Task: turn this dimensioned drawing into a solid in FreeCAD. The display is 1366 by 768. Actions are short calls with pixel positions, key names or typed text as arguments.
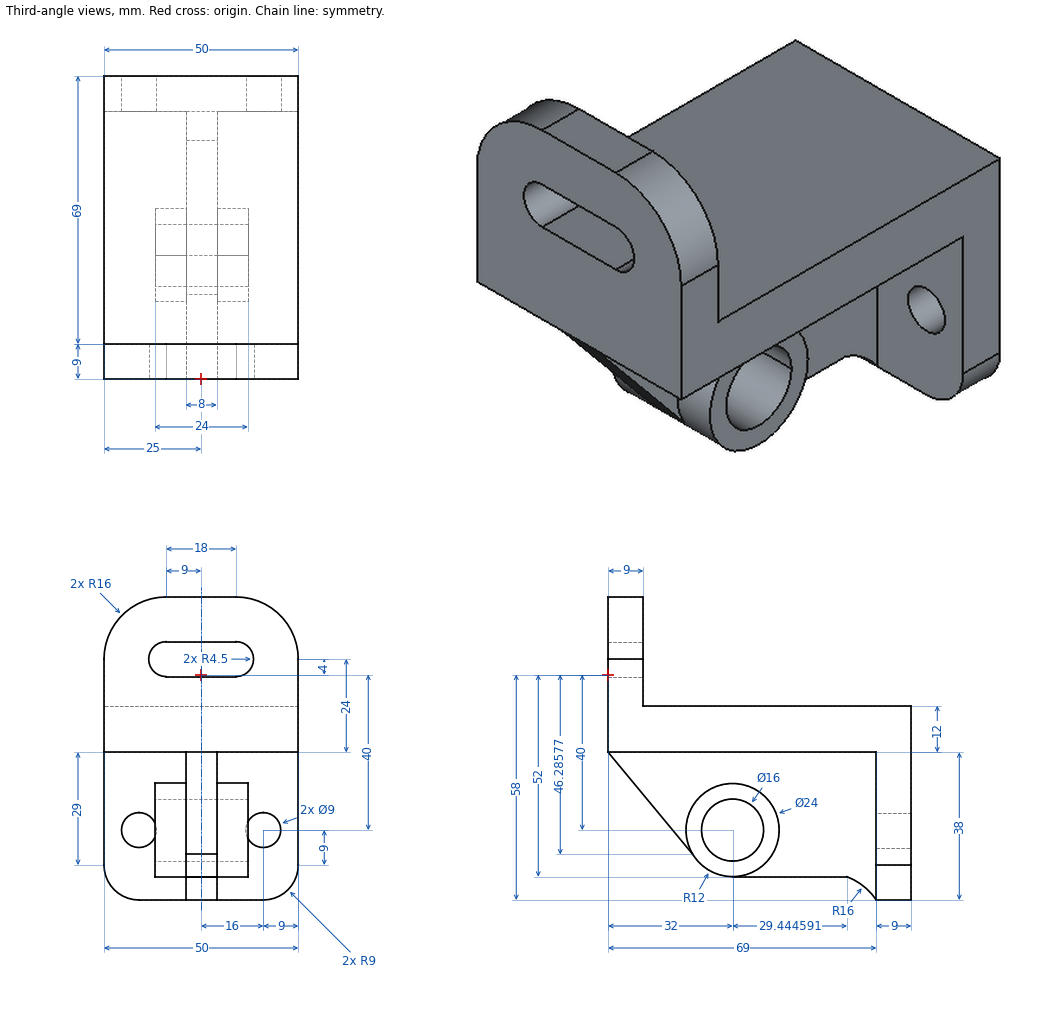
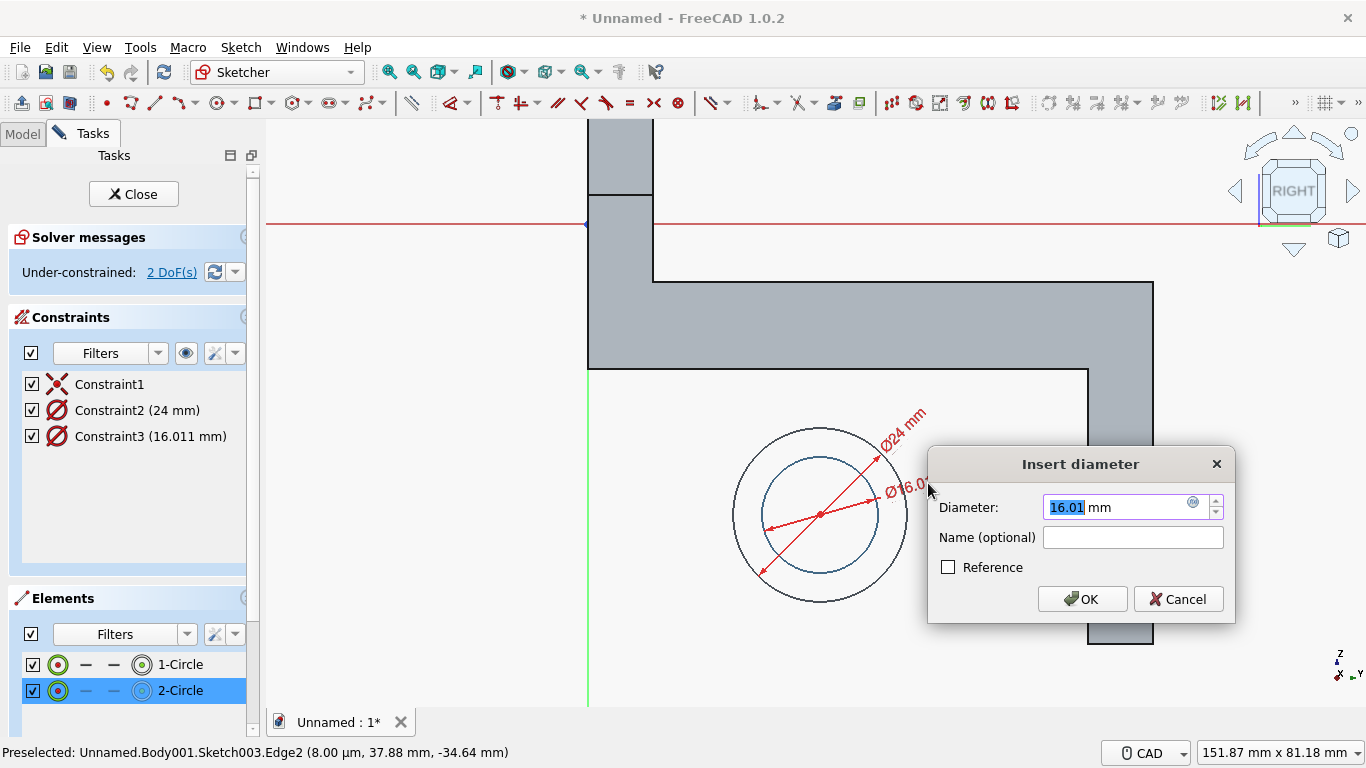
text(16)
key(Return)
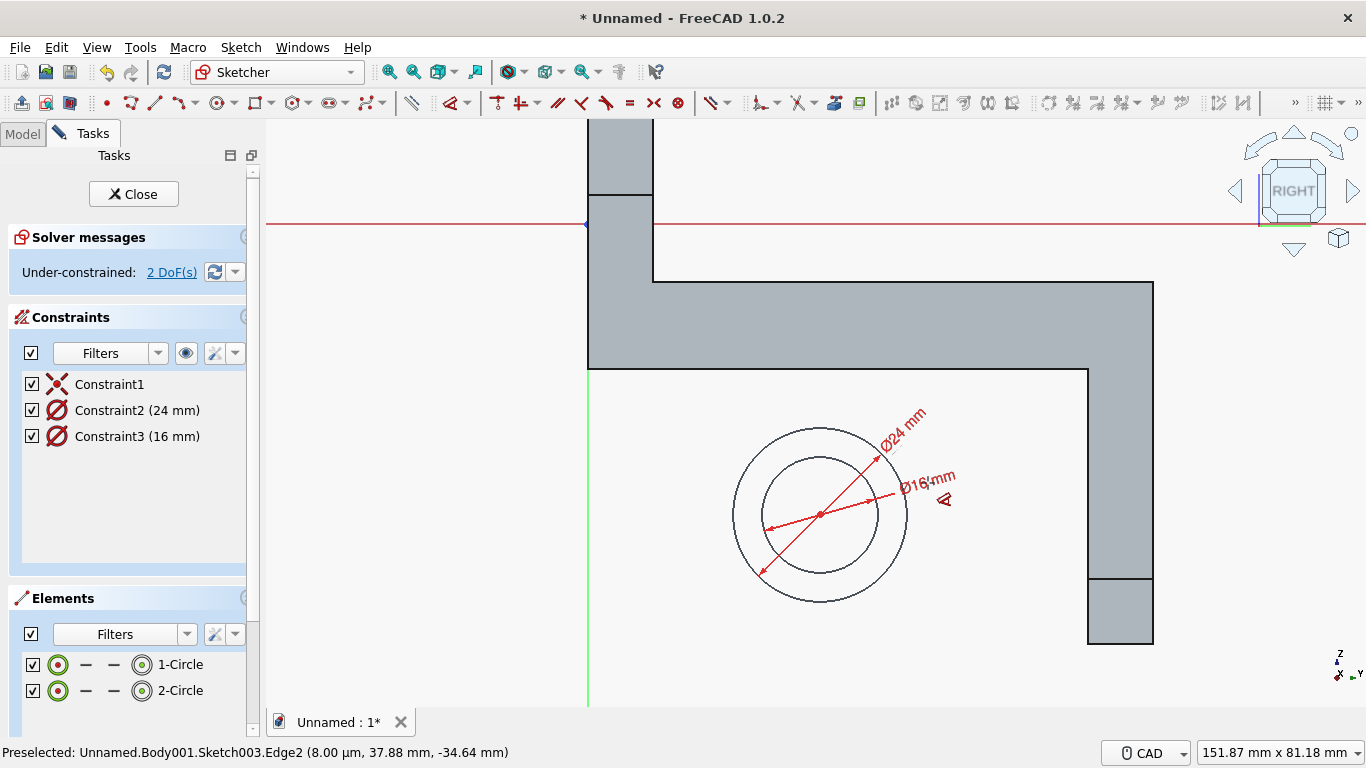
click(820, 515)
click(704, 190)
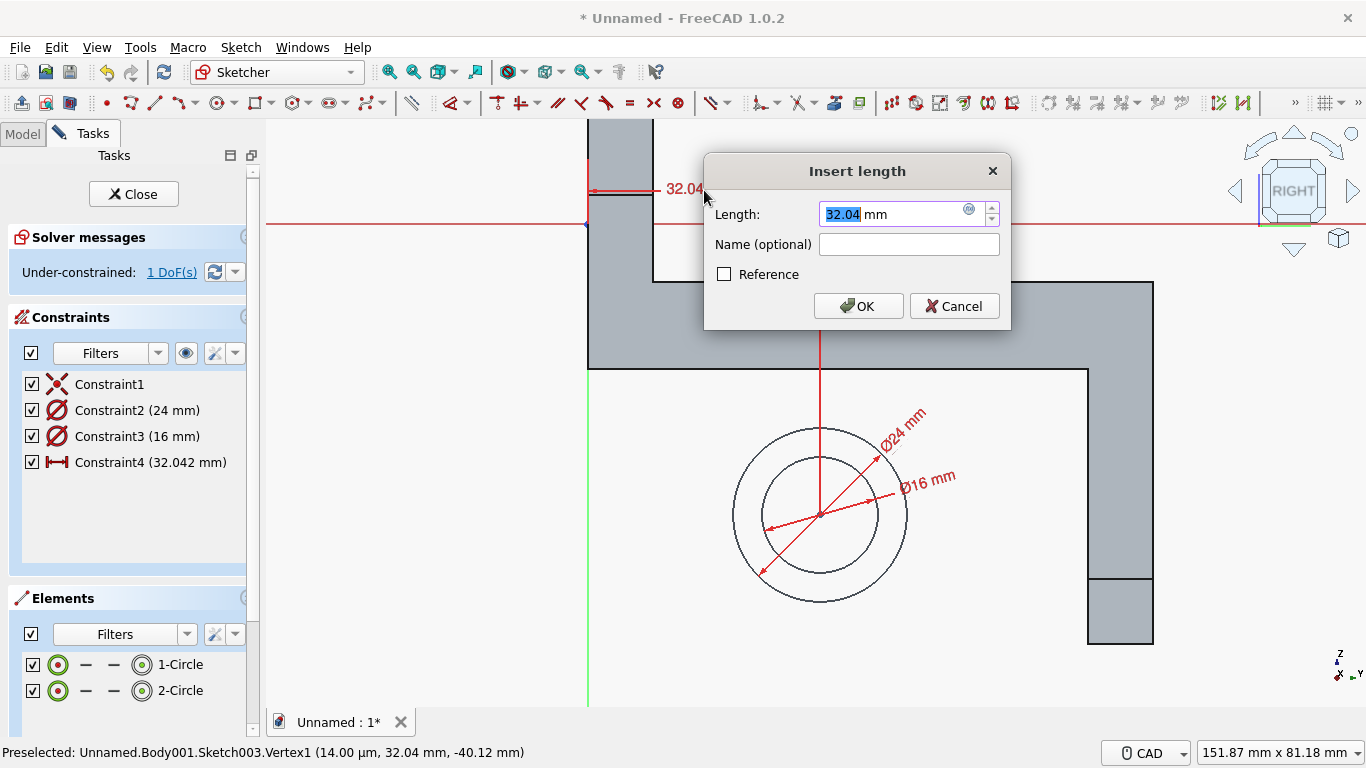
text(32)
key(Return)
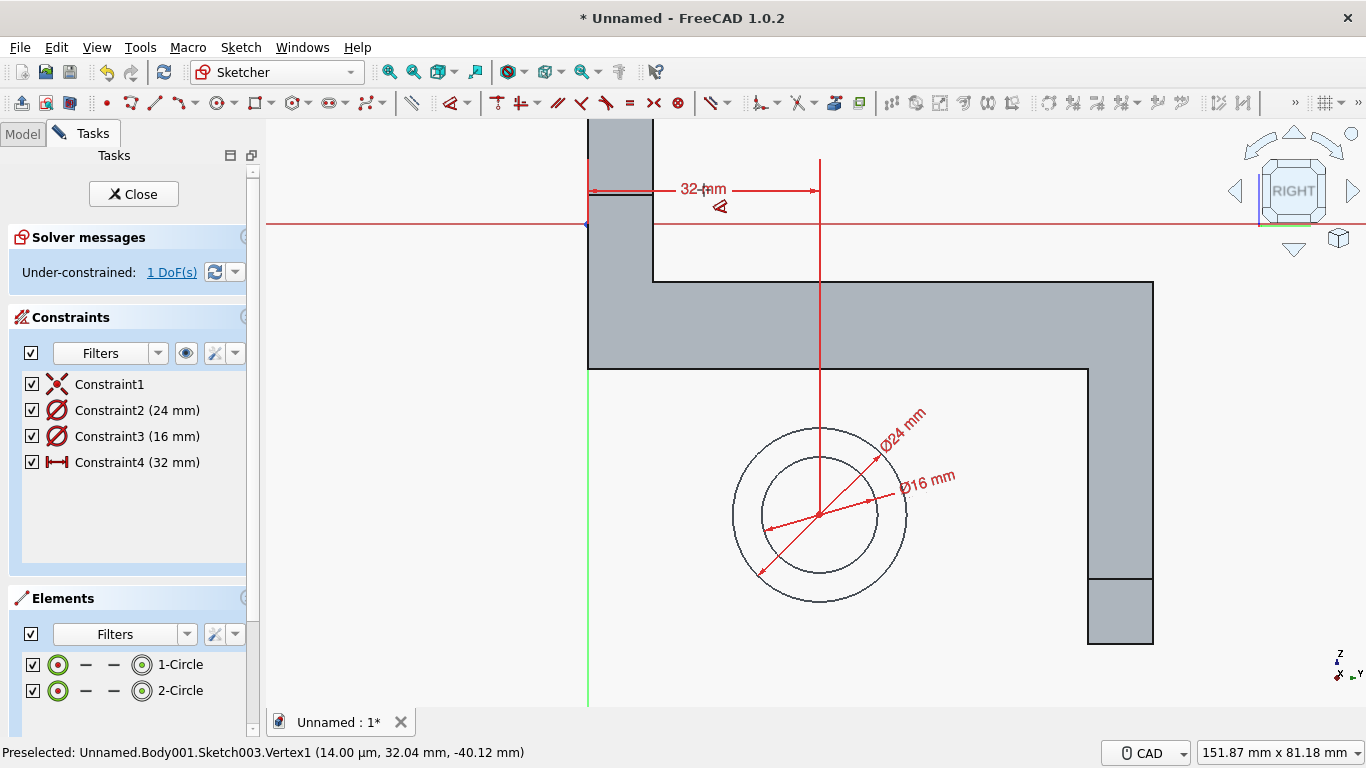
click(820, 515)
click(554, 370)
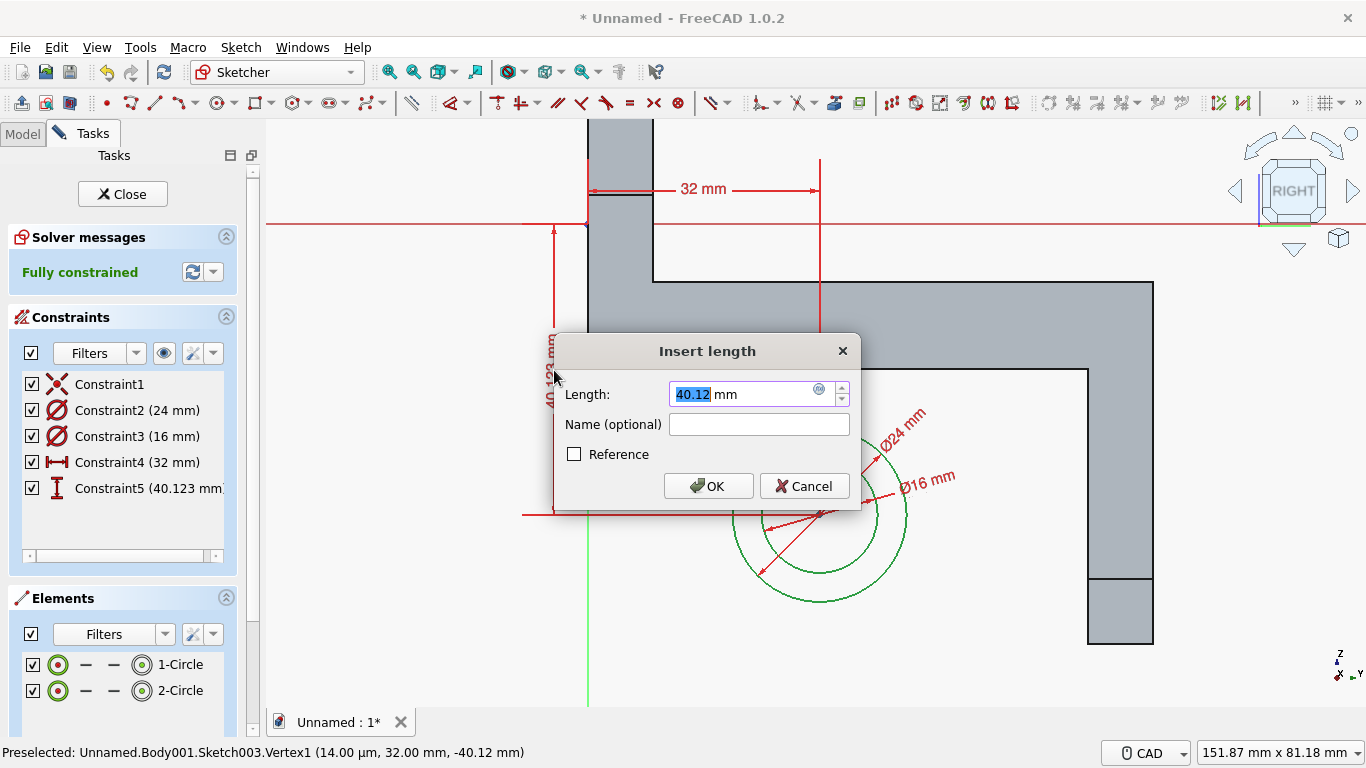
text(40)
key(Return)
key(Escape)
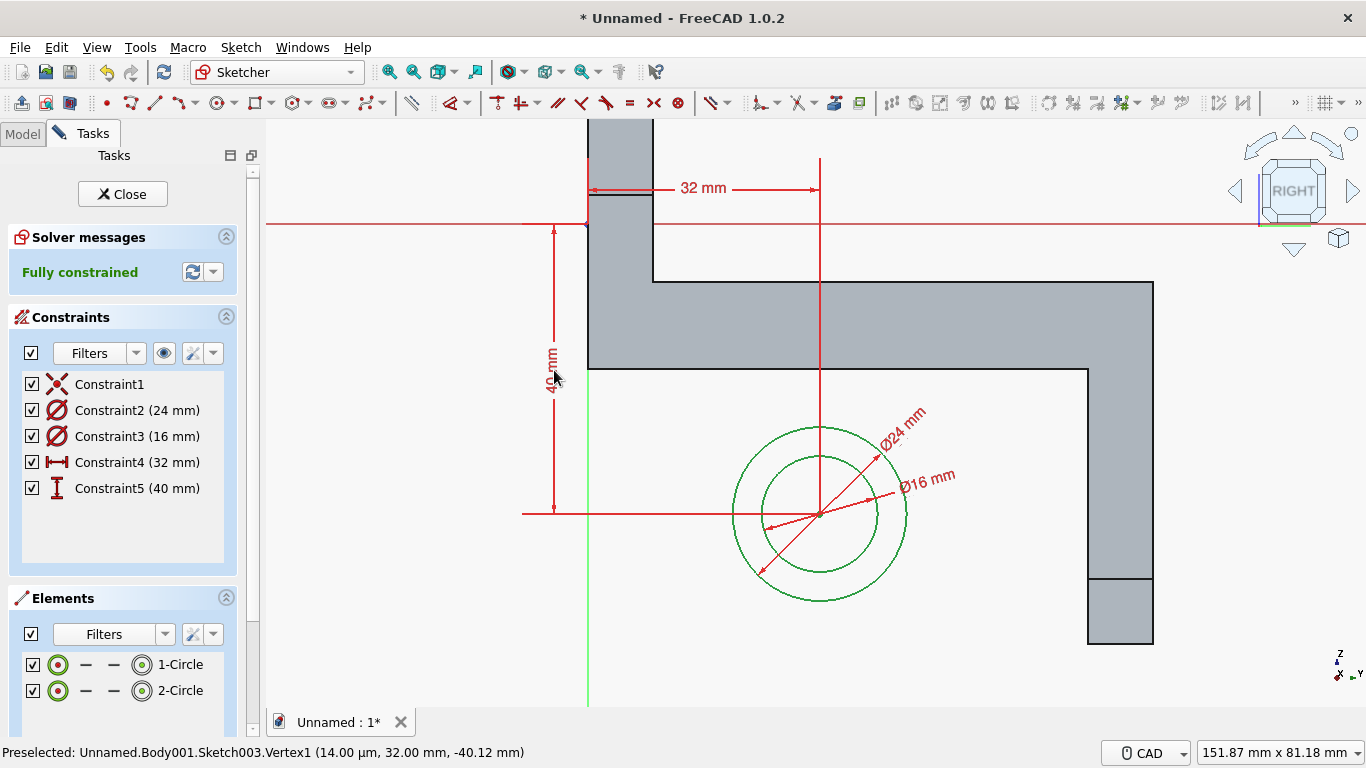
click(123, 194)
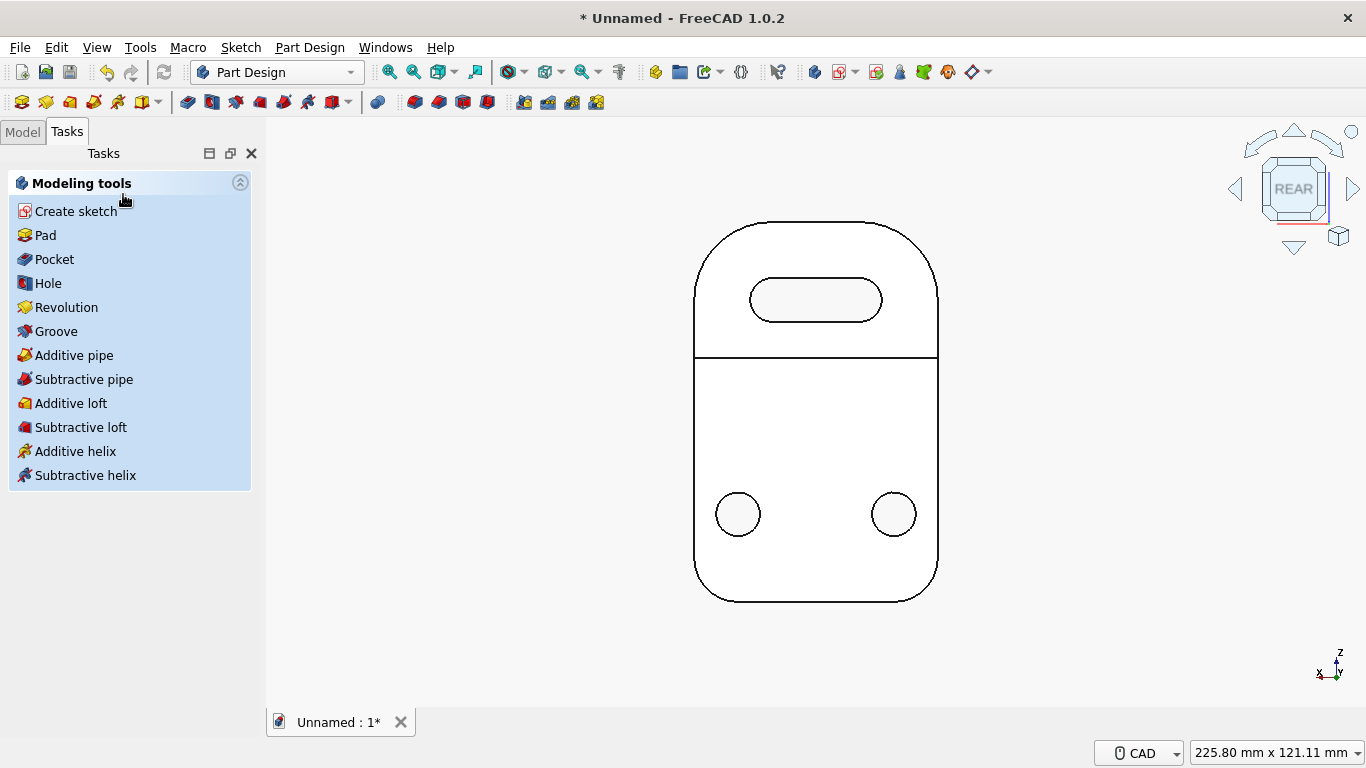
click(22, 102)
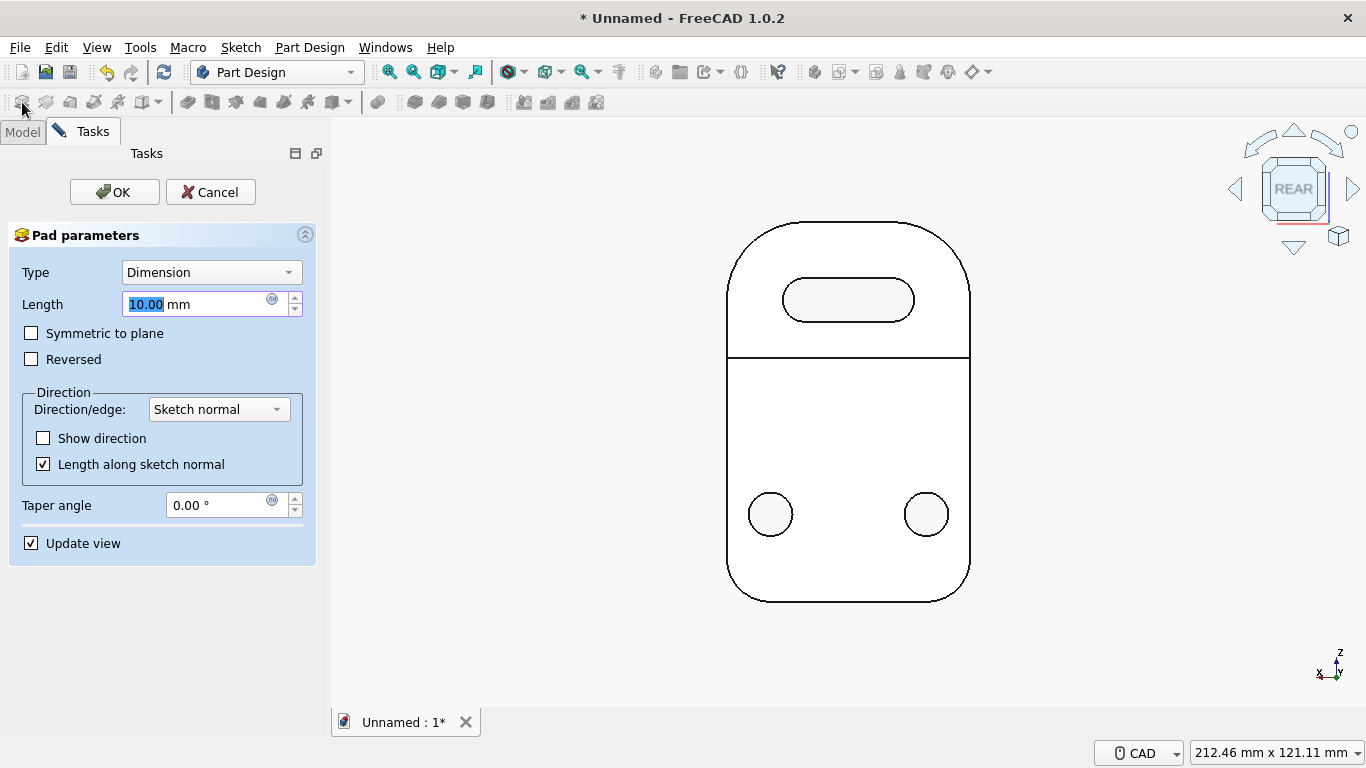
text(24)
key(Tab)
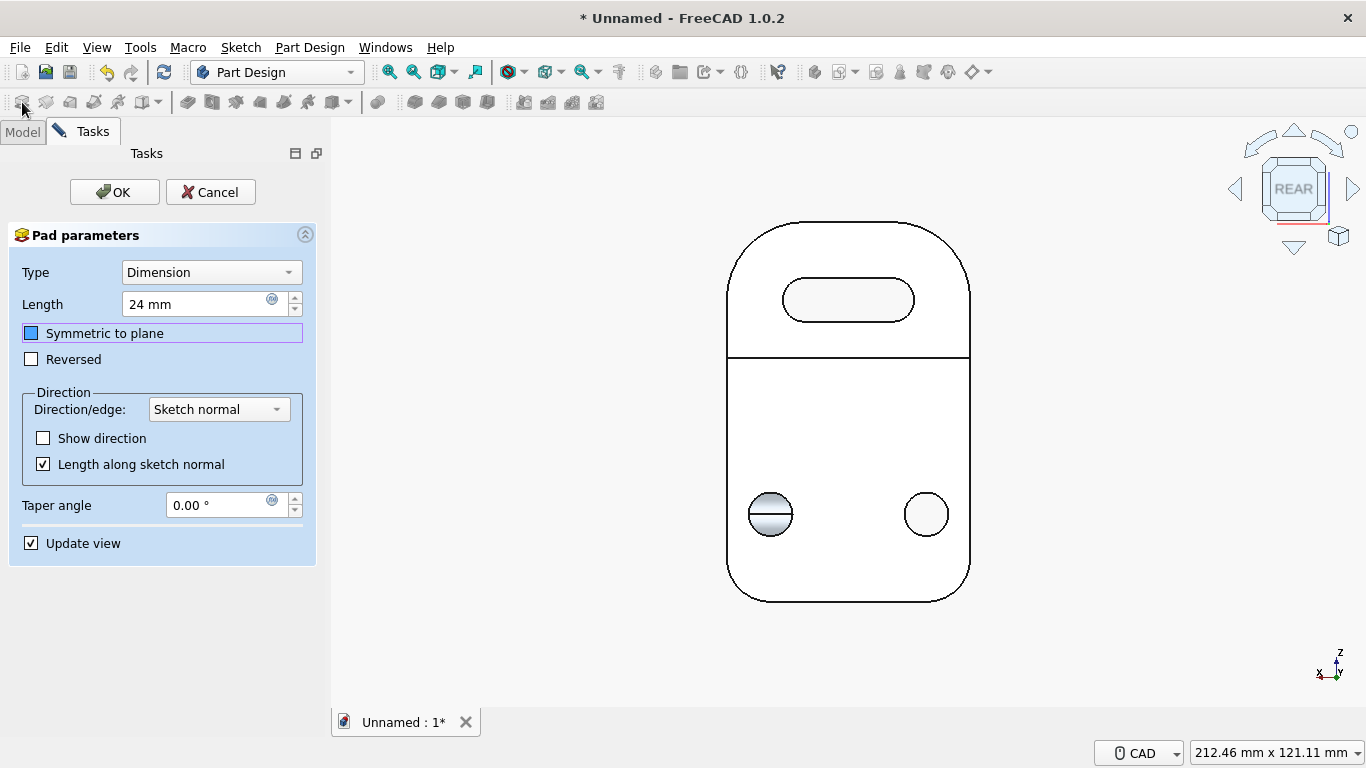
click(30, 333)